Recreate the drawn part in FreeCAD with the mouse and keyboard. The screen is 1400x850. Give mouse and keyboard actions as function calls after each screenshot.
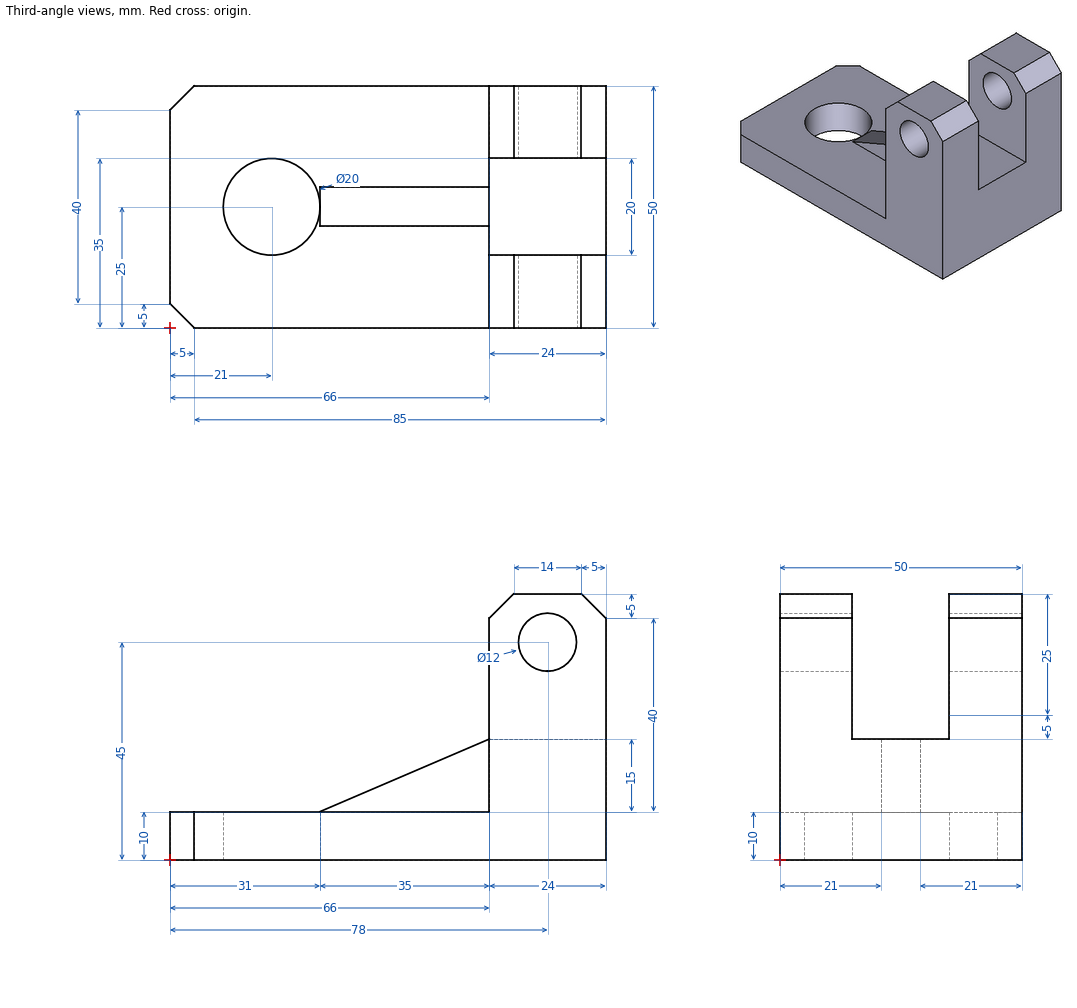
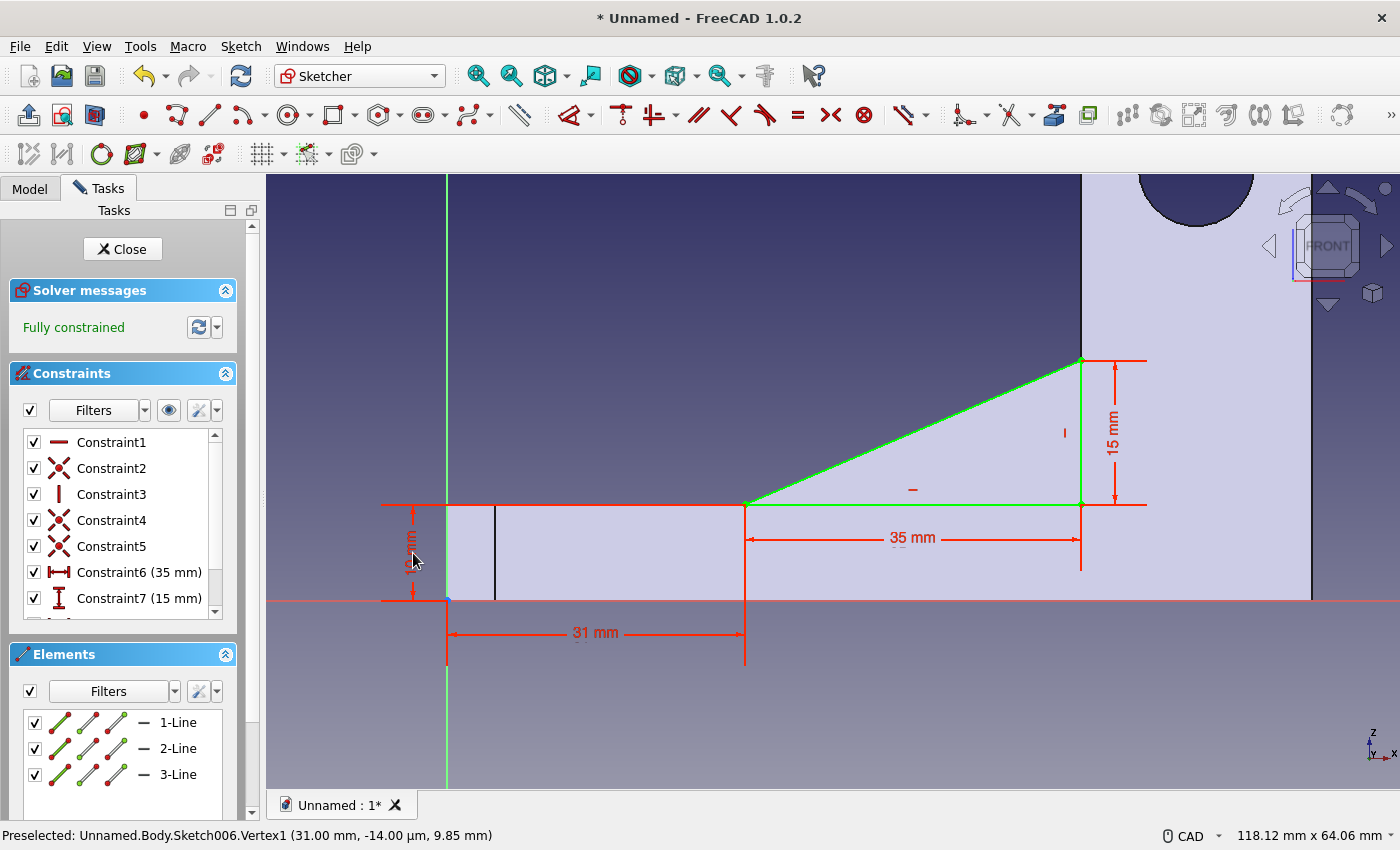
click(123, 249)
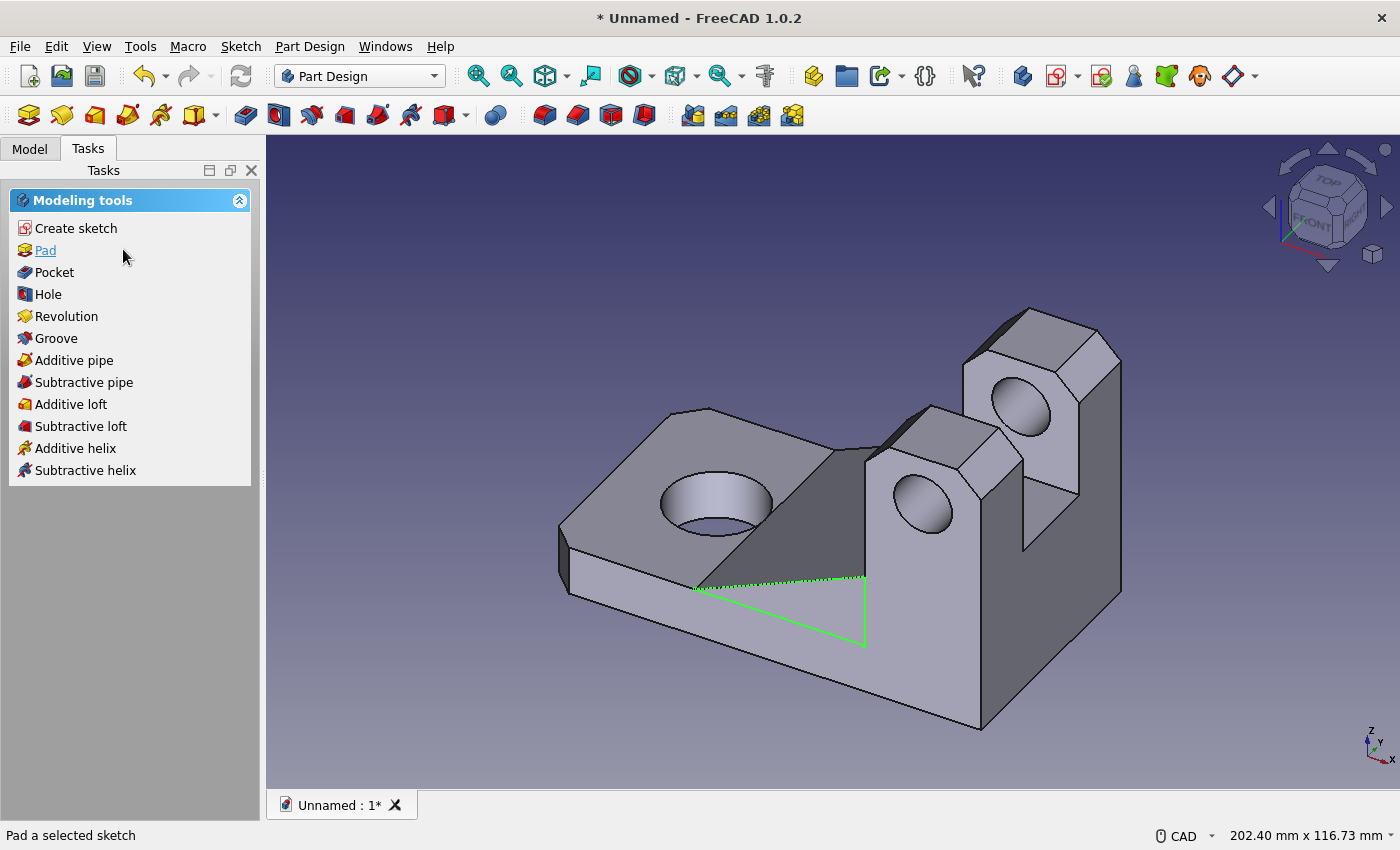
click(246, 116)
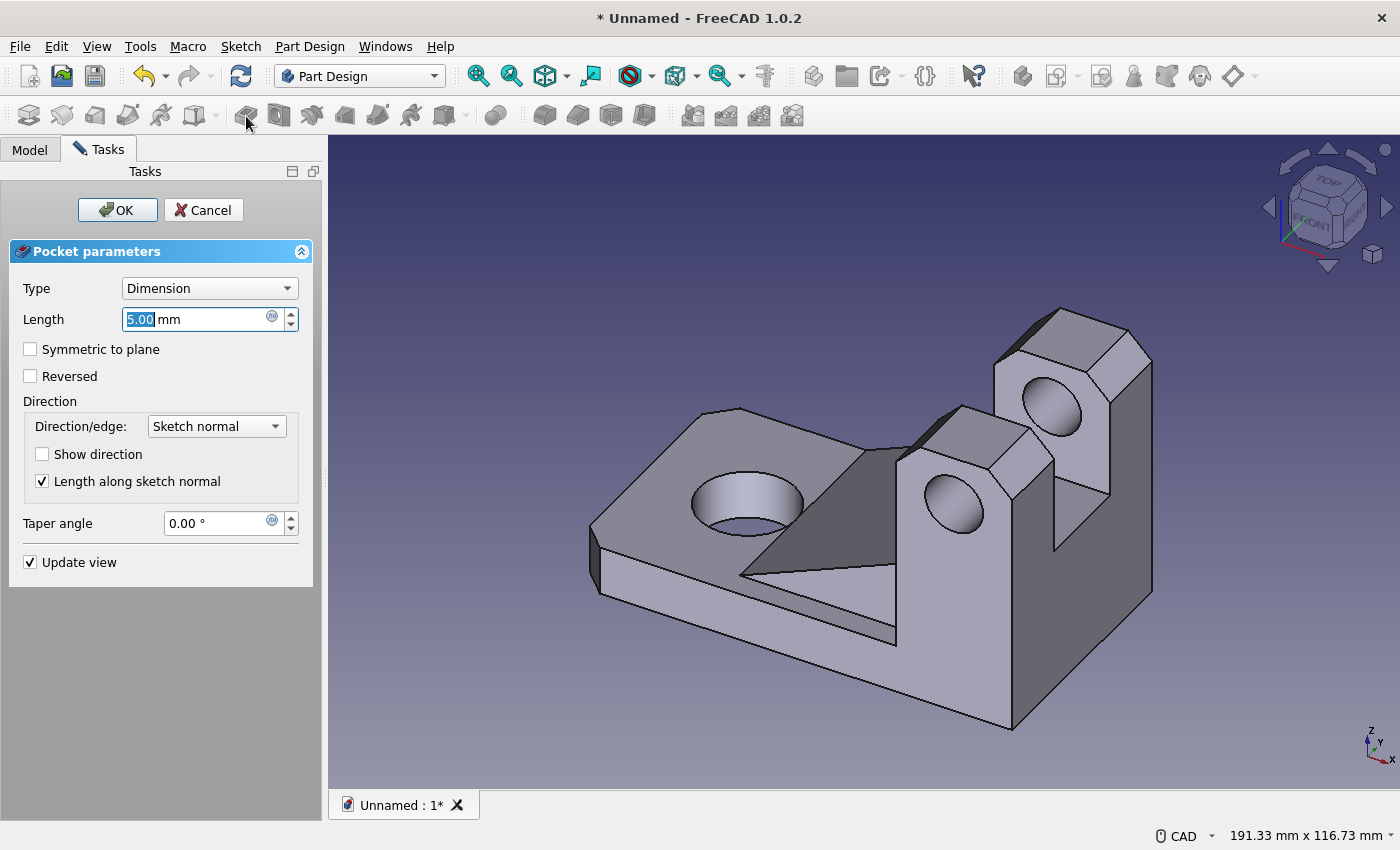
text(21)
key(Tab)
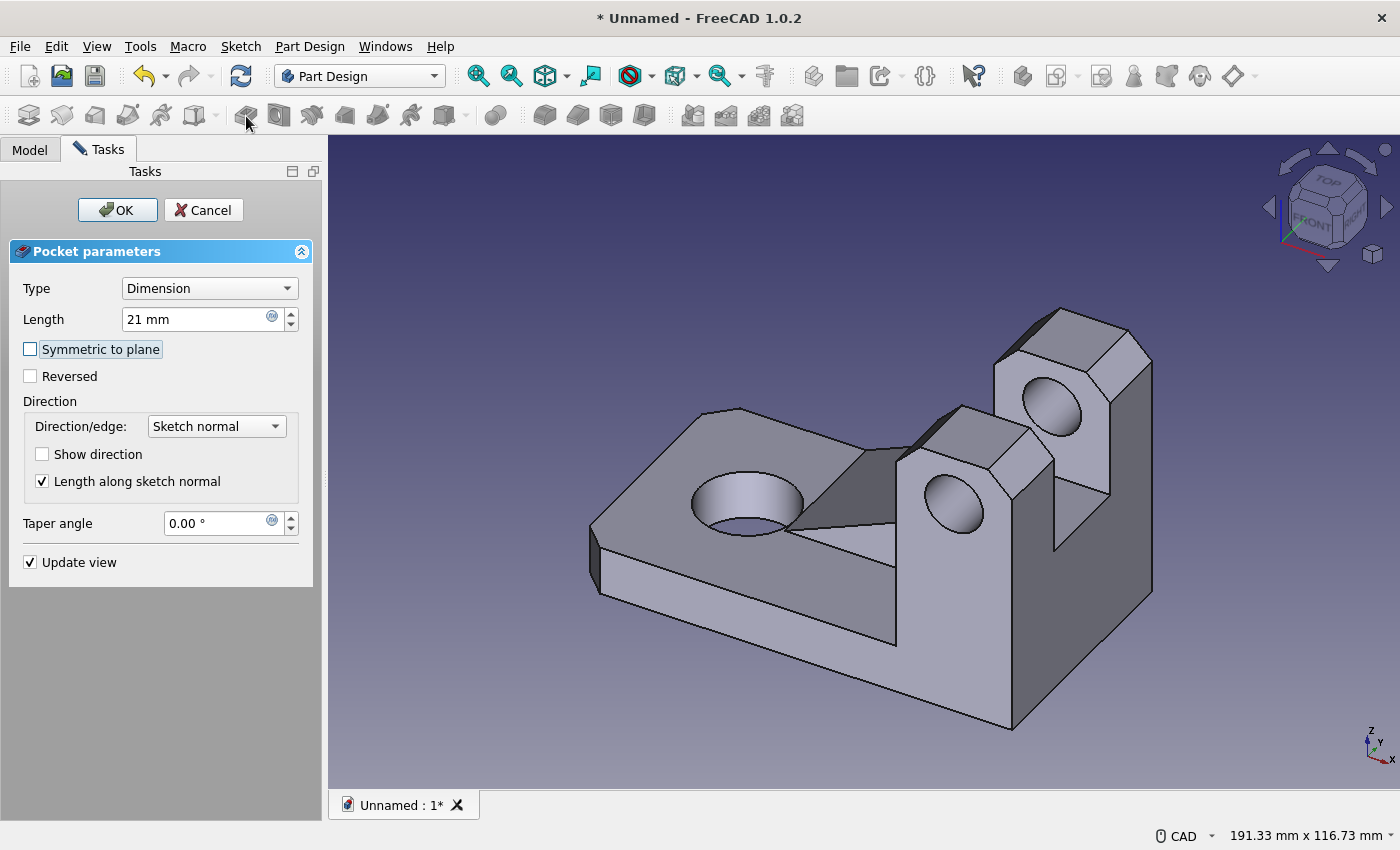
click(118, 210)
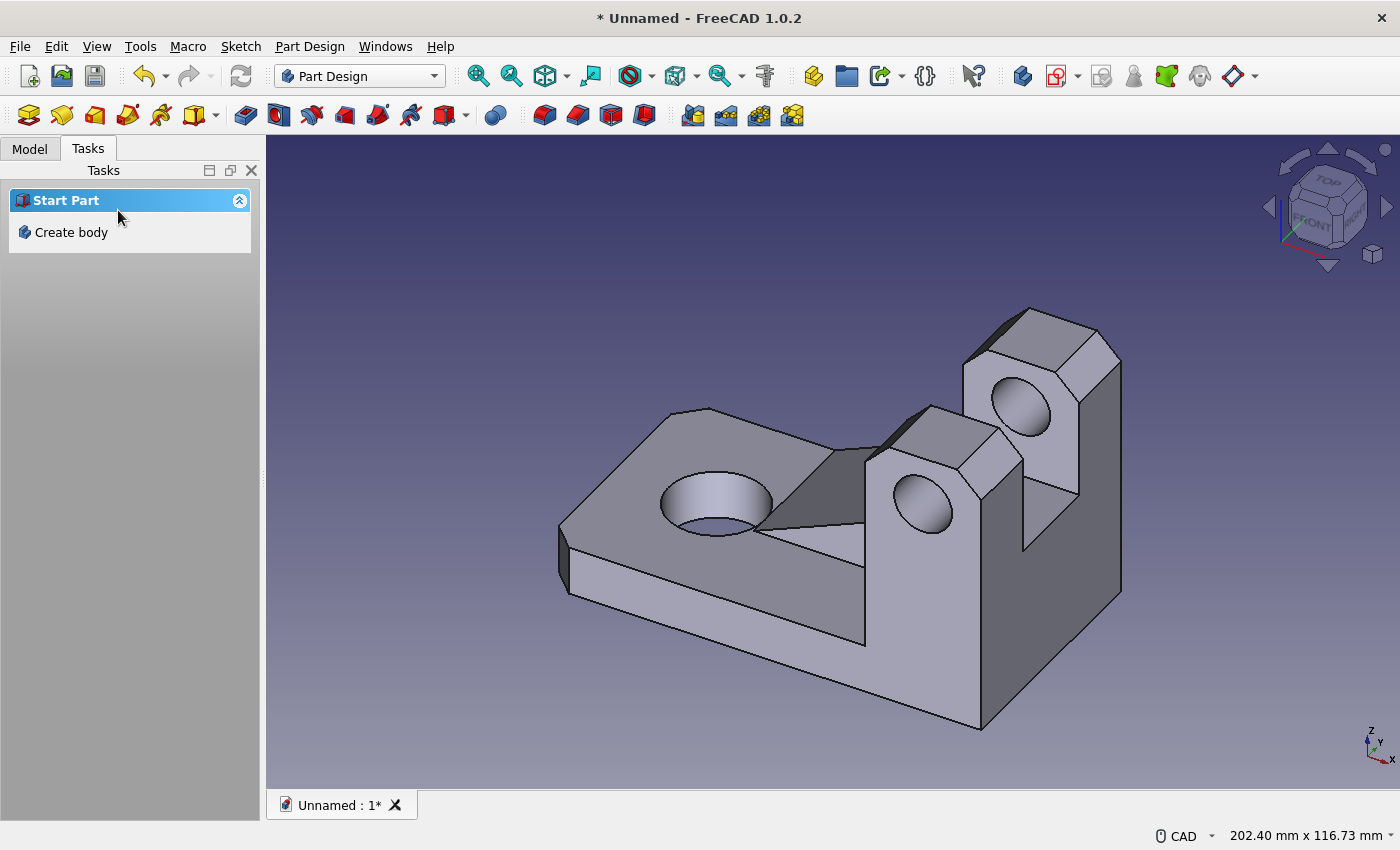
key(4)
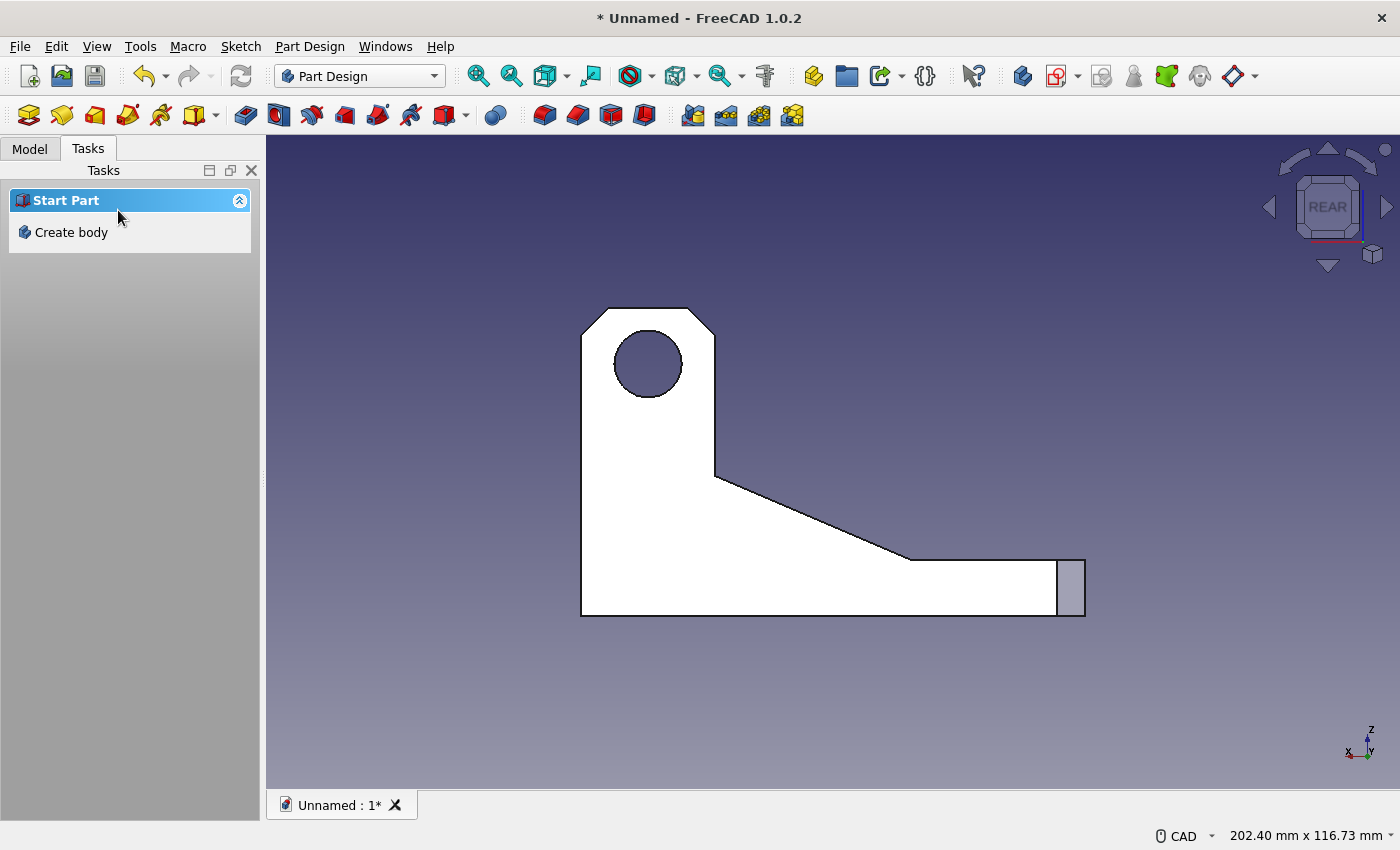
click(683, 549)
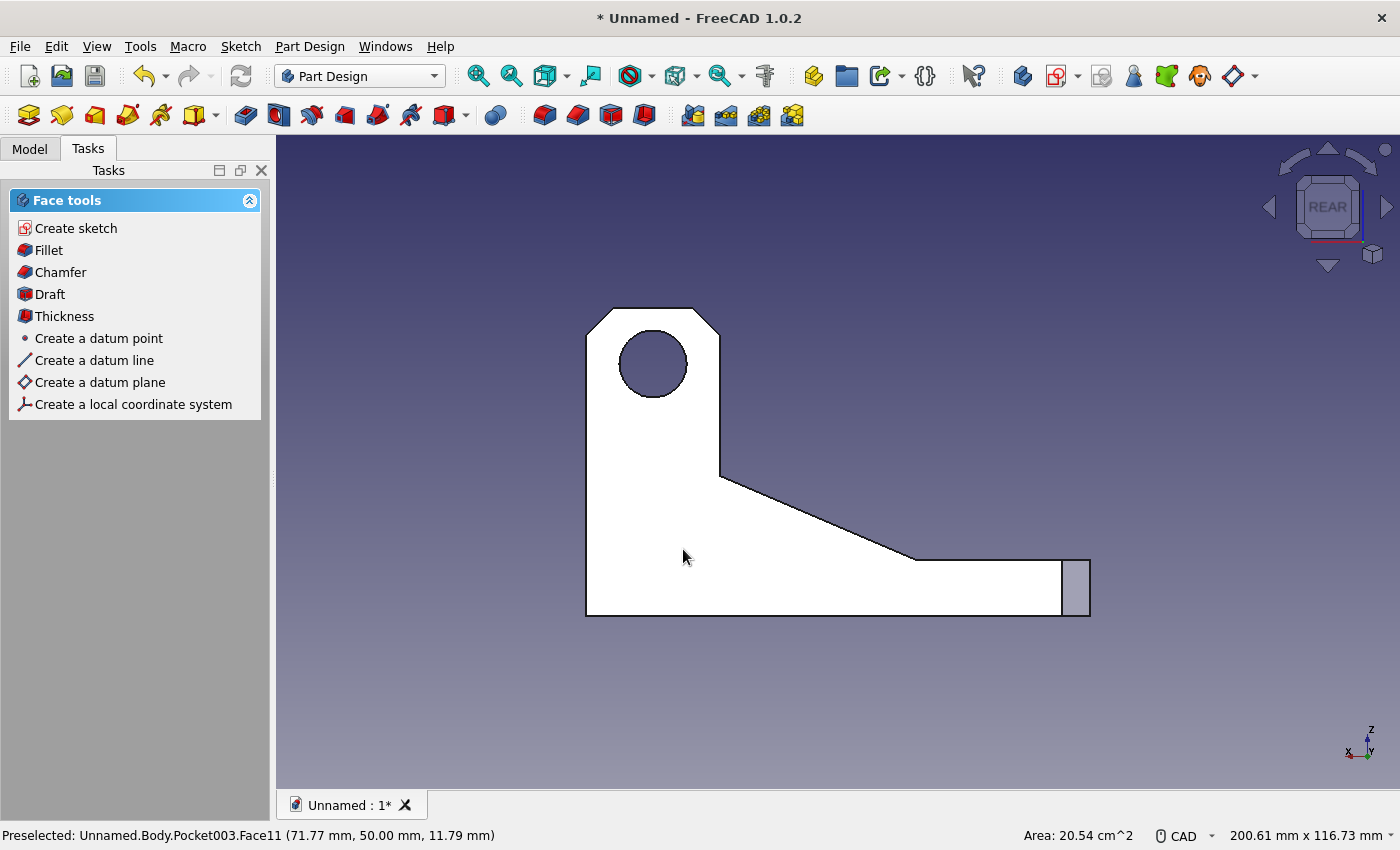
click(1056, 76)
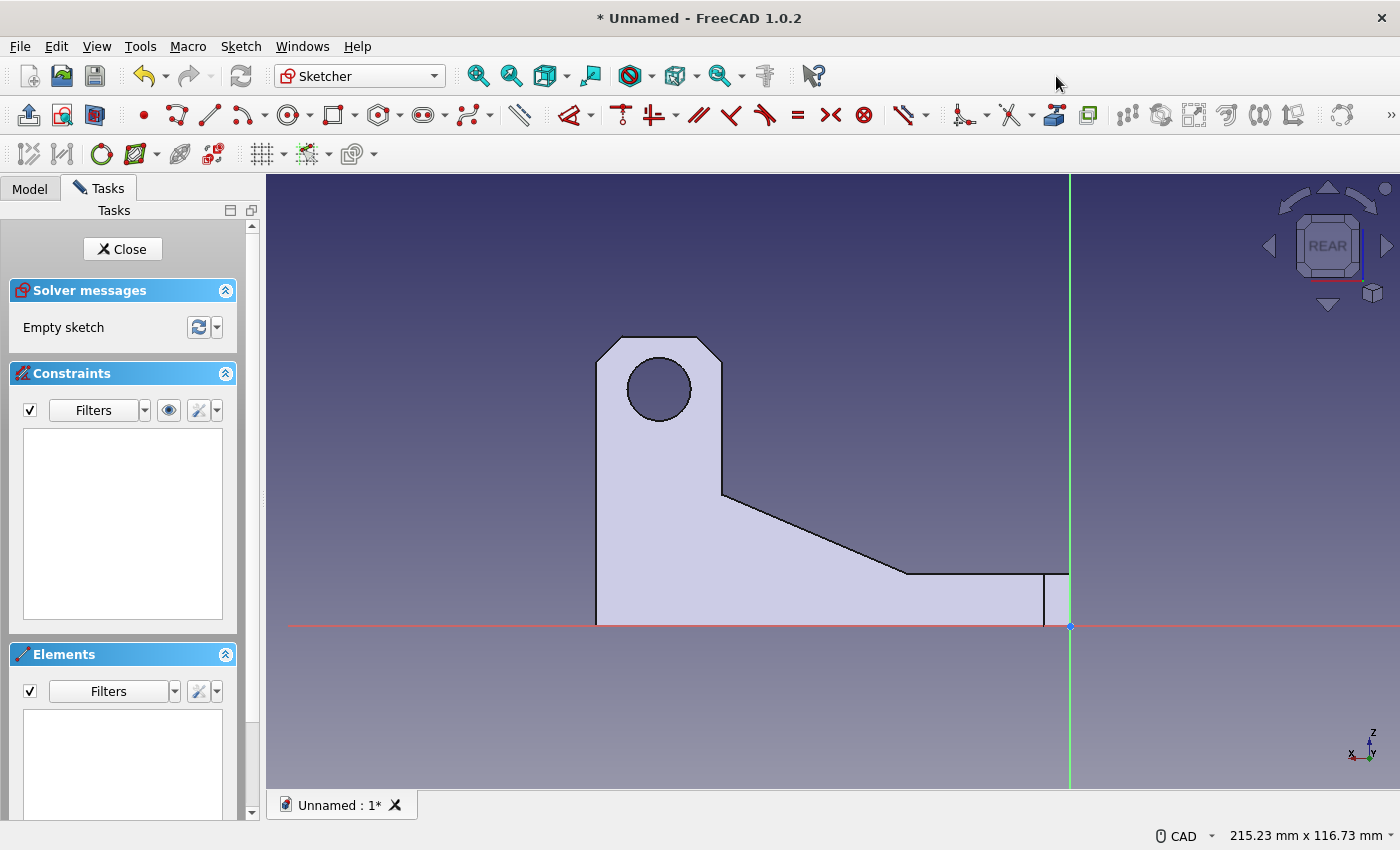
scroll(1056, 657, up, 3)